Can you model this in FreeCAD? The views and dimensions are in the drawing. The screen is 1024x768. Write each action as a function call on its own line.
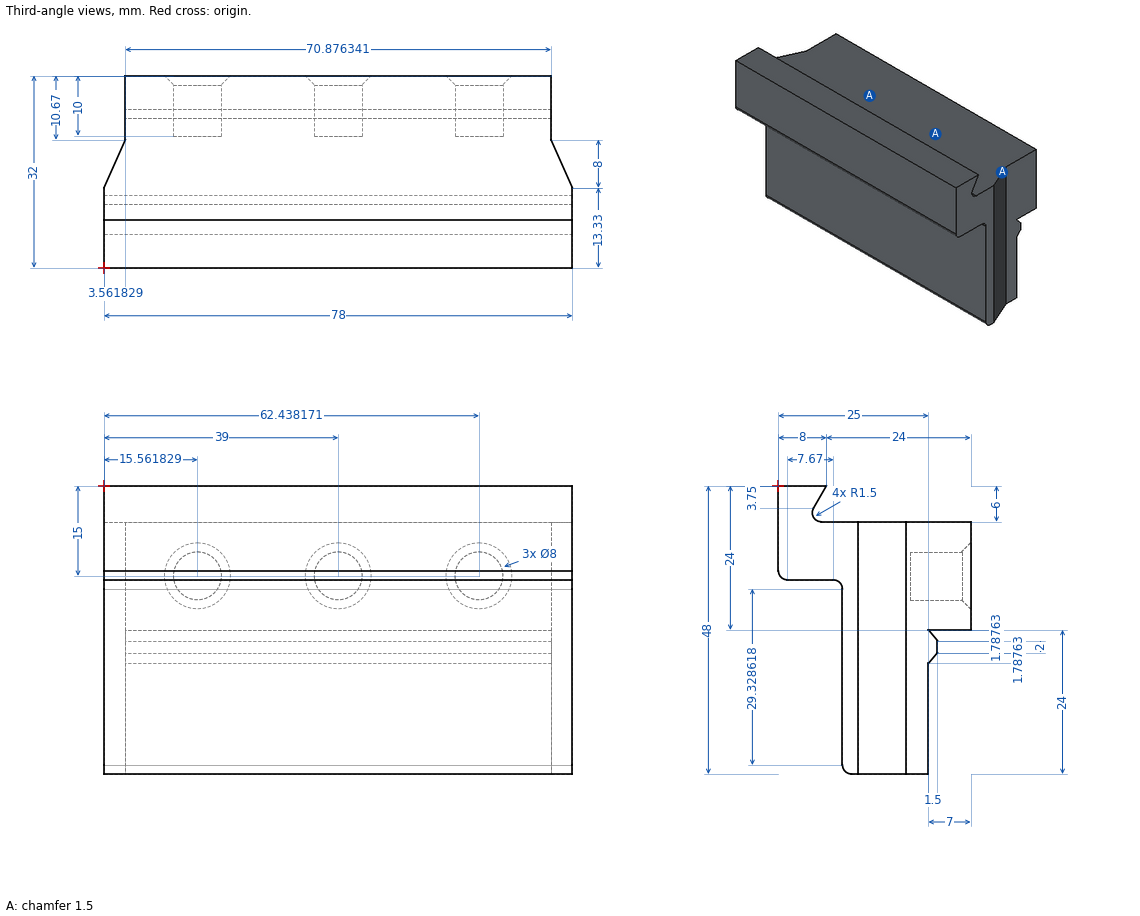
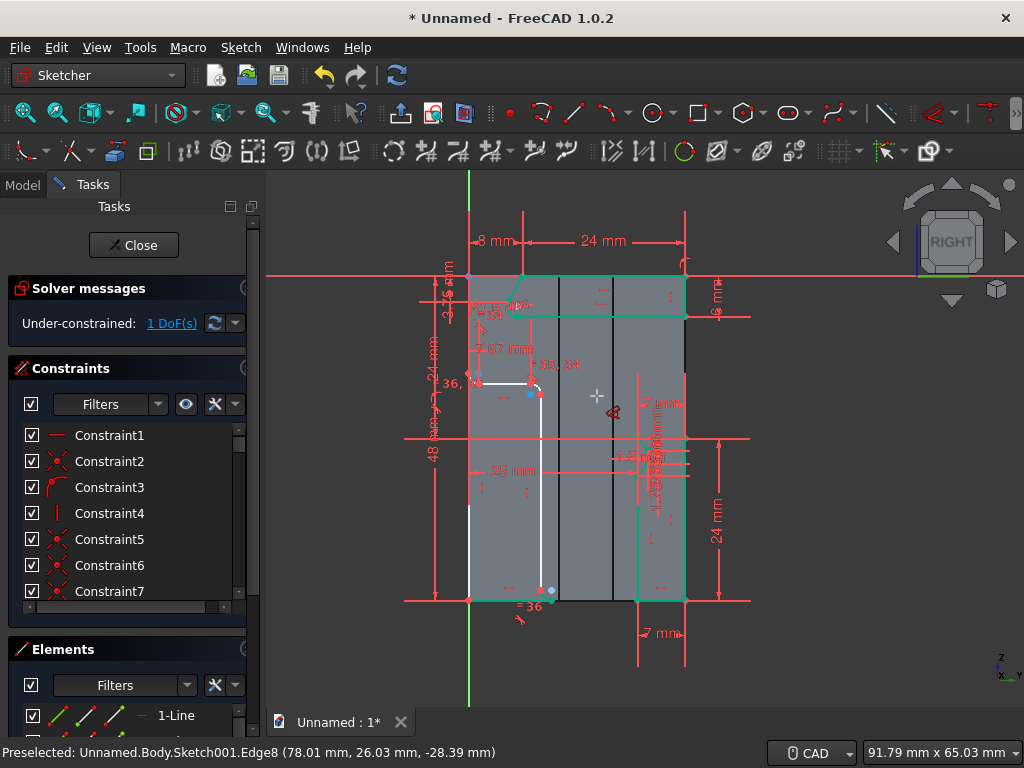
click(541, 453)
click(507, 447)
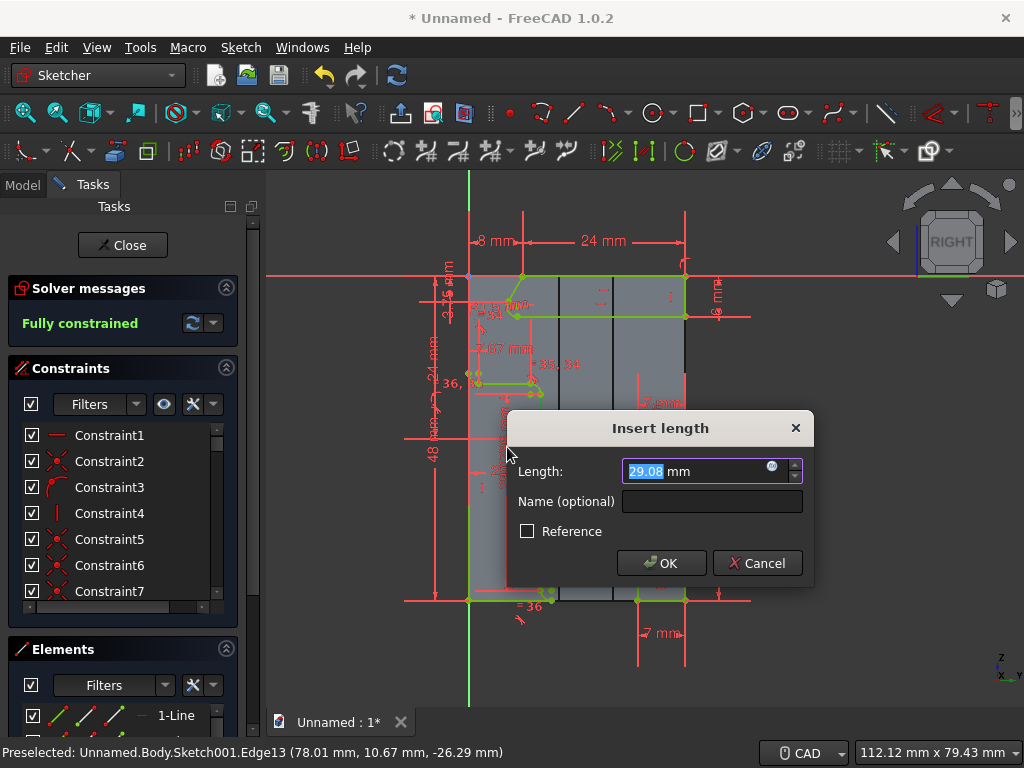
text(29.328618)
key(Return)
key(Escape)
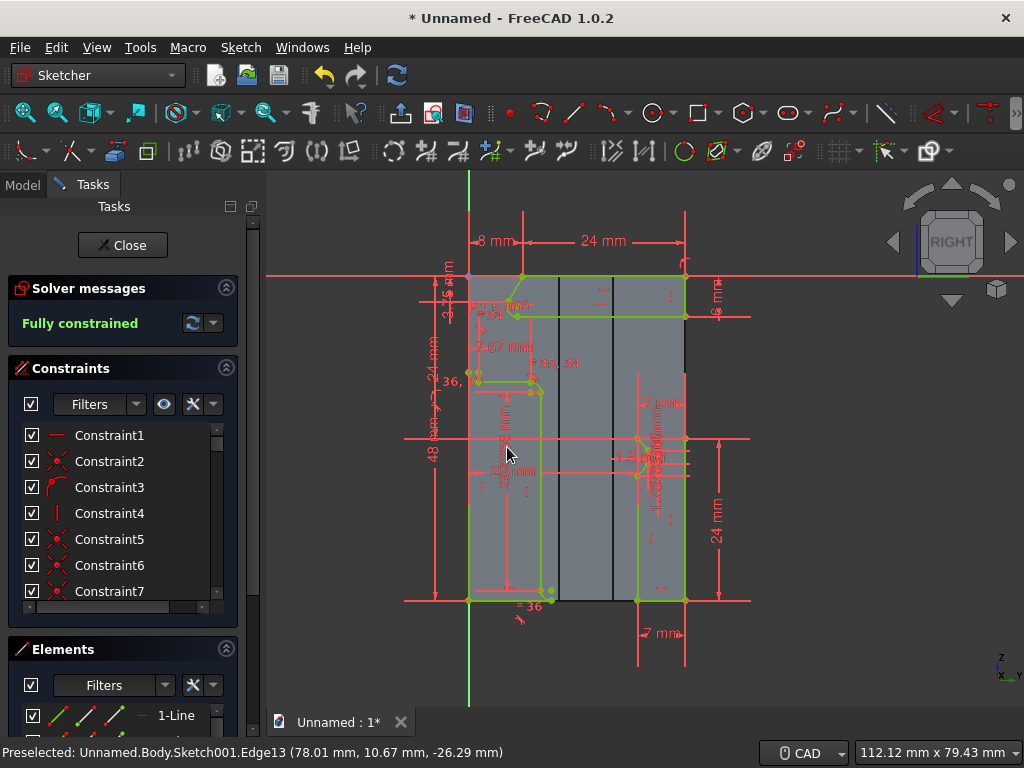
click(123, 245)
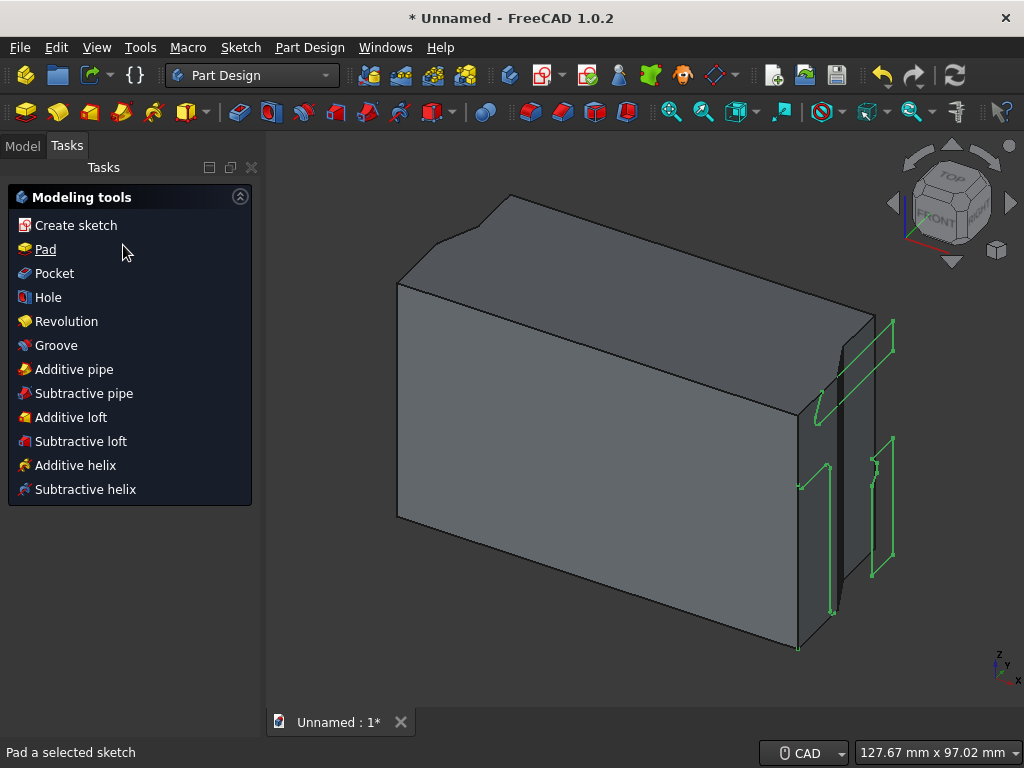
click(240, 112)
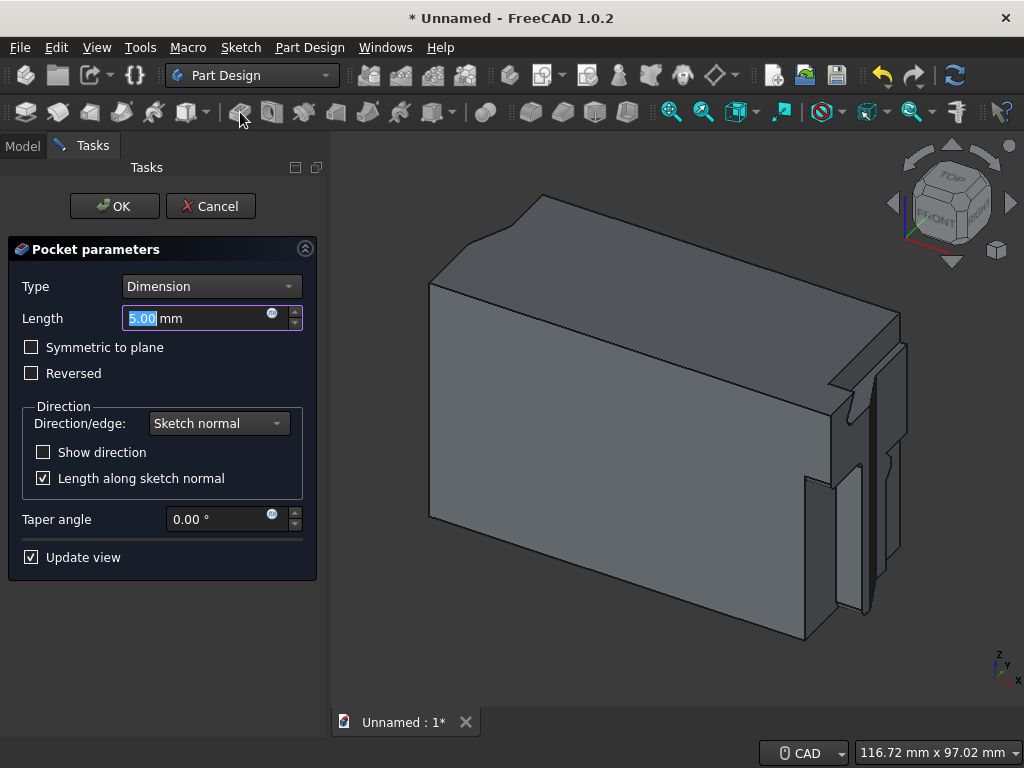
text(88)
key(Tab)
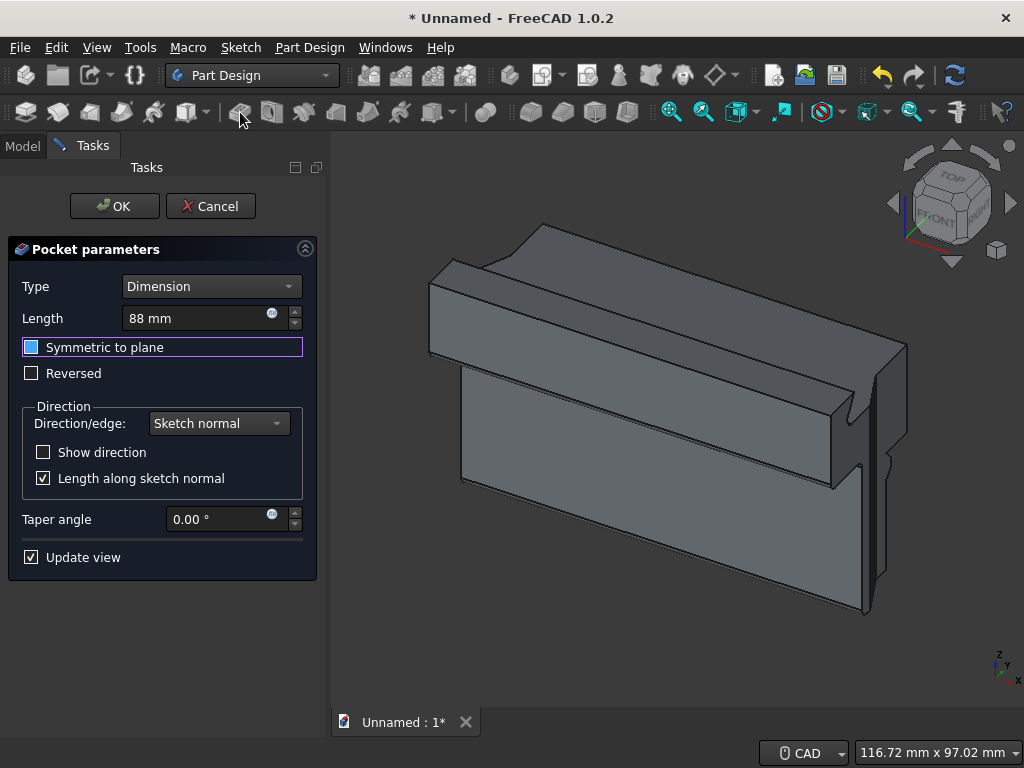
click(115, 206)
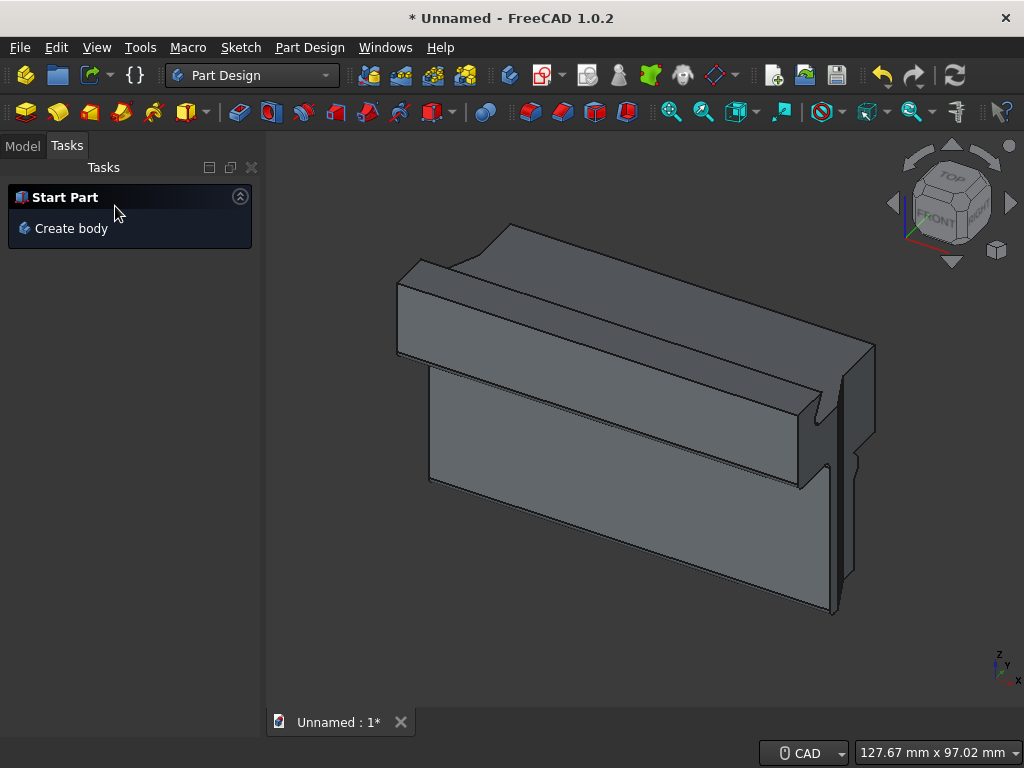
key(4)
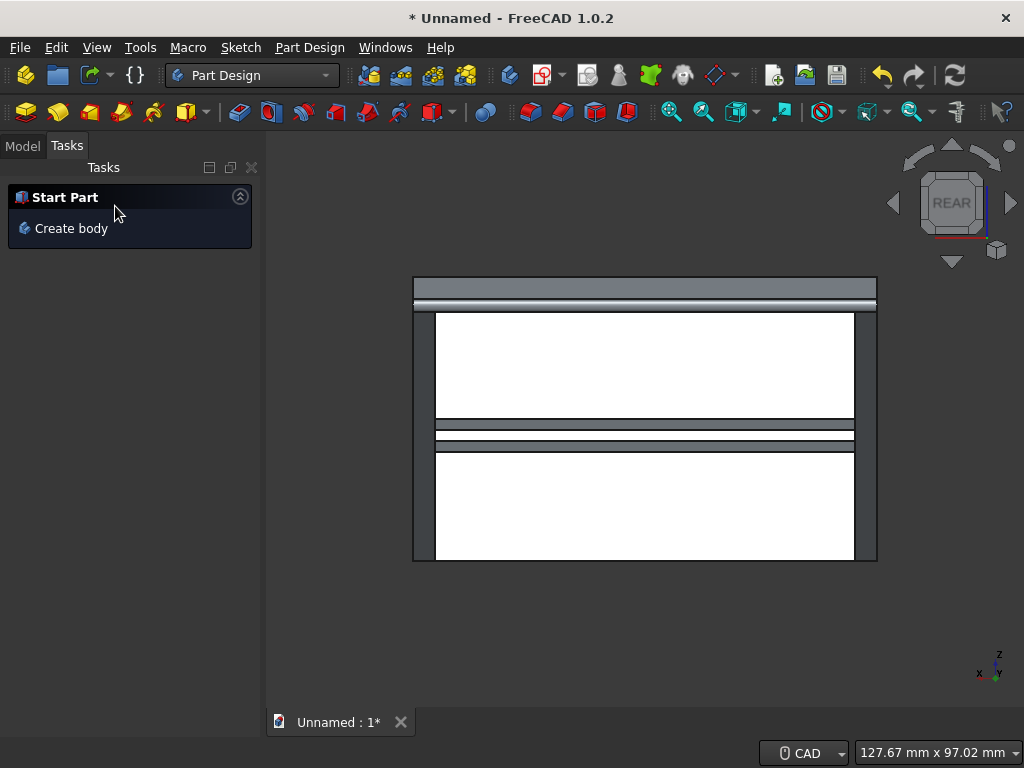
click(525, 365)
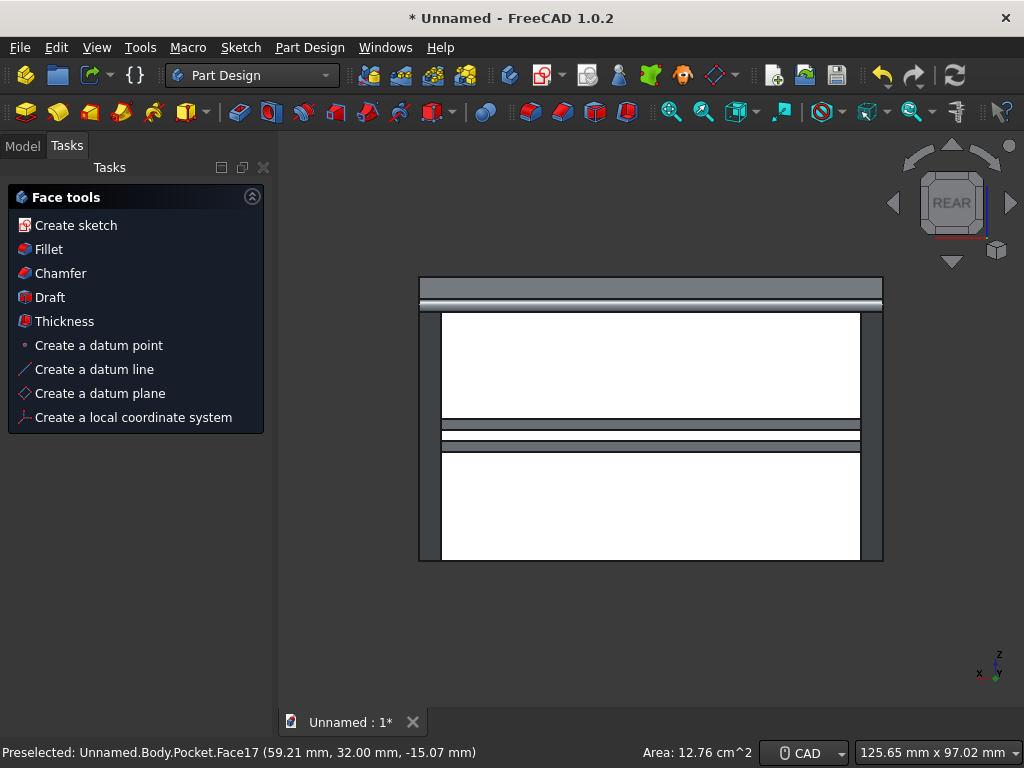
click(542, 76)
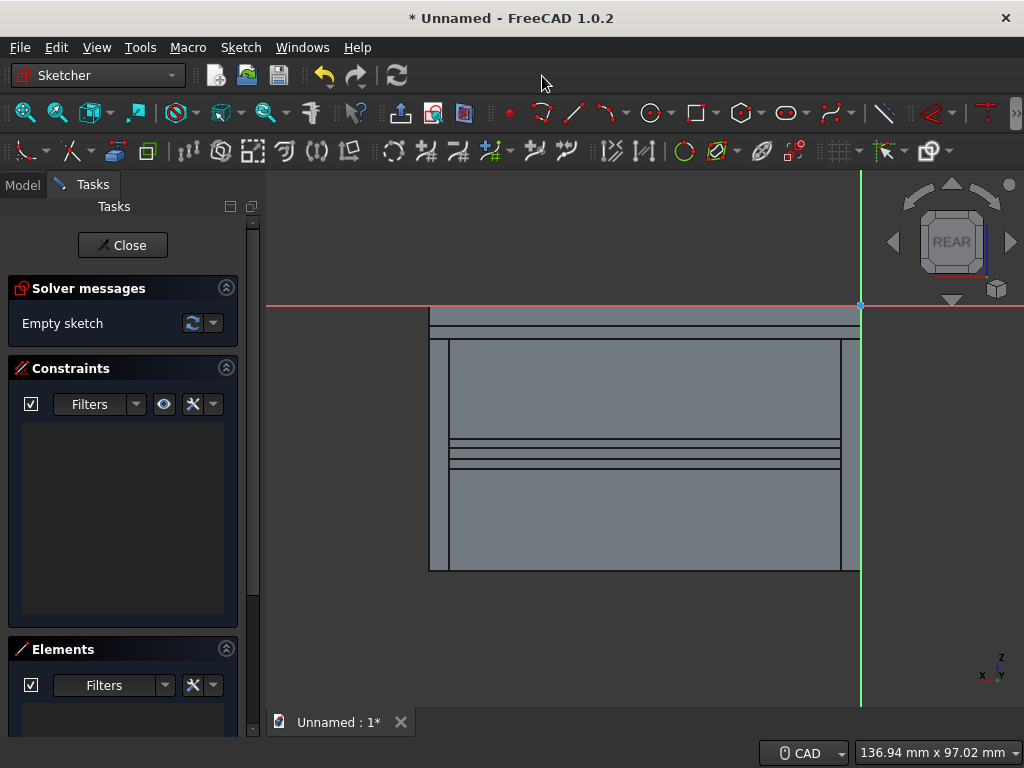
scroll(294, 679, down, 1)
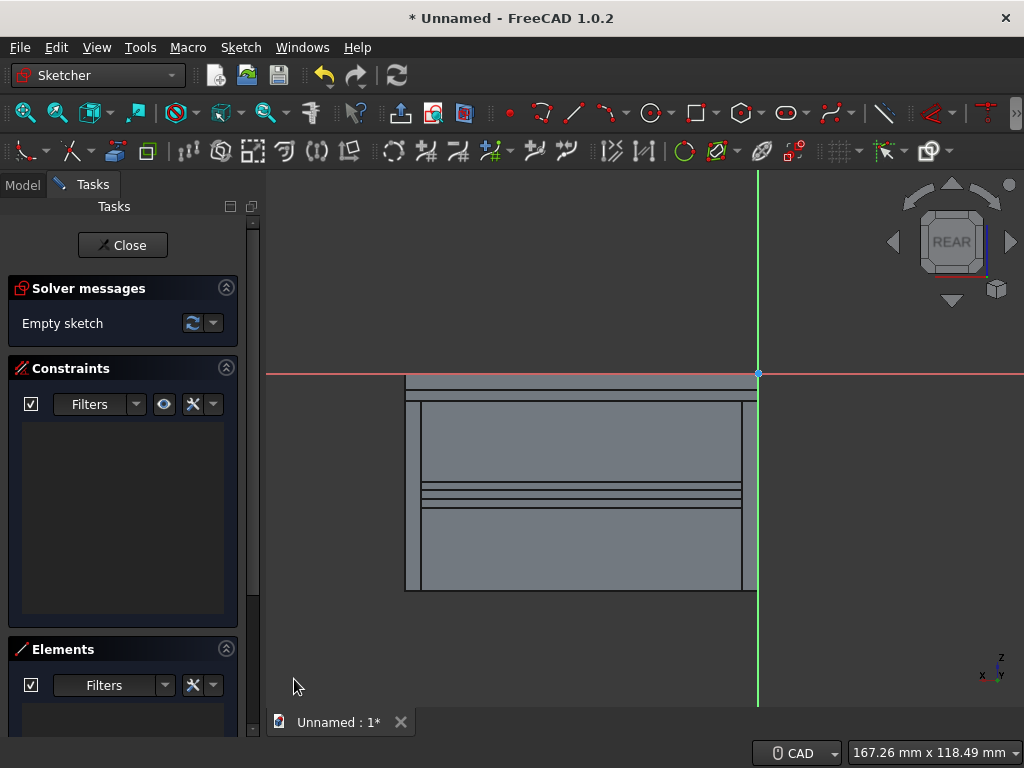
click(652, 114)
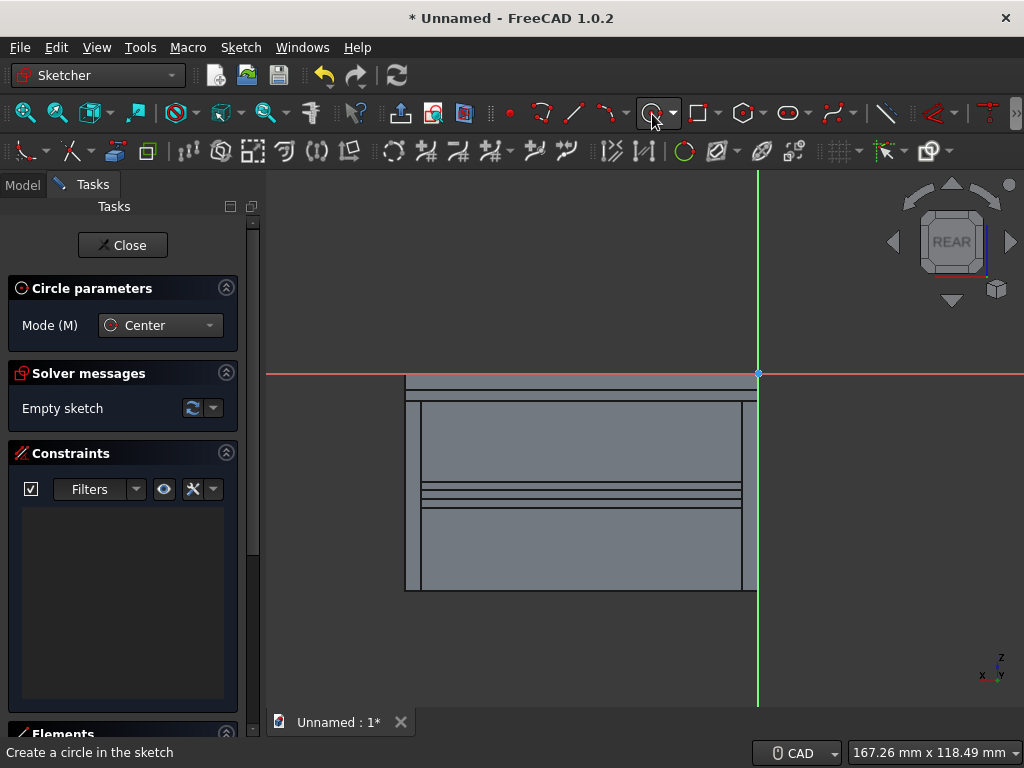
scroll(475, 441, up, 2)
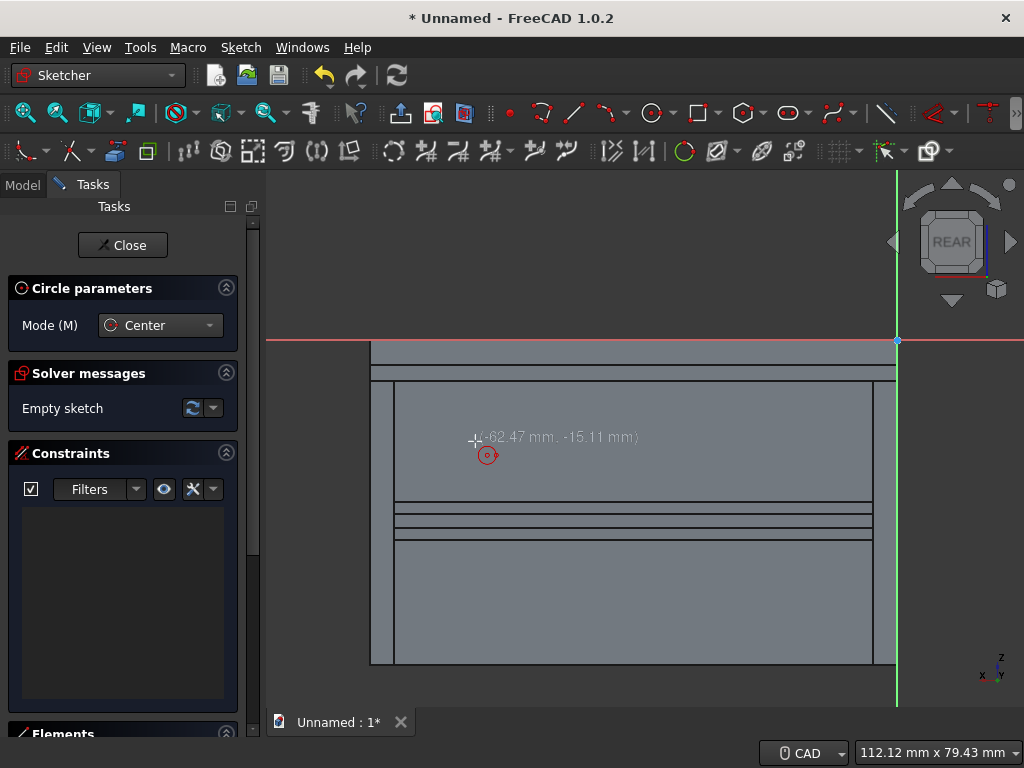
click(475, 441)
move(494, 422)